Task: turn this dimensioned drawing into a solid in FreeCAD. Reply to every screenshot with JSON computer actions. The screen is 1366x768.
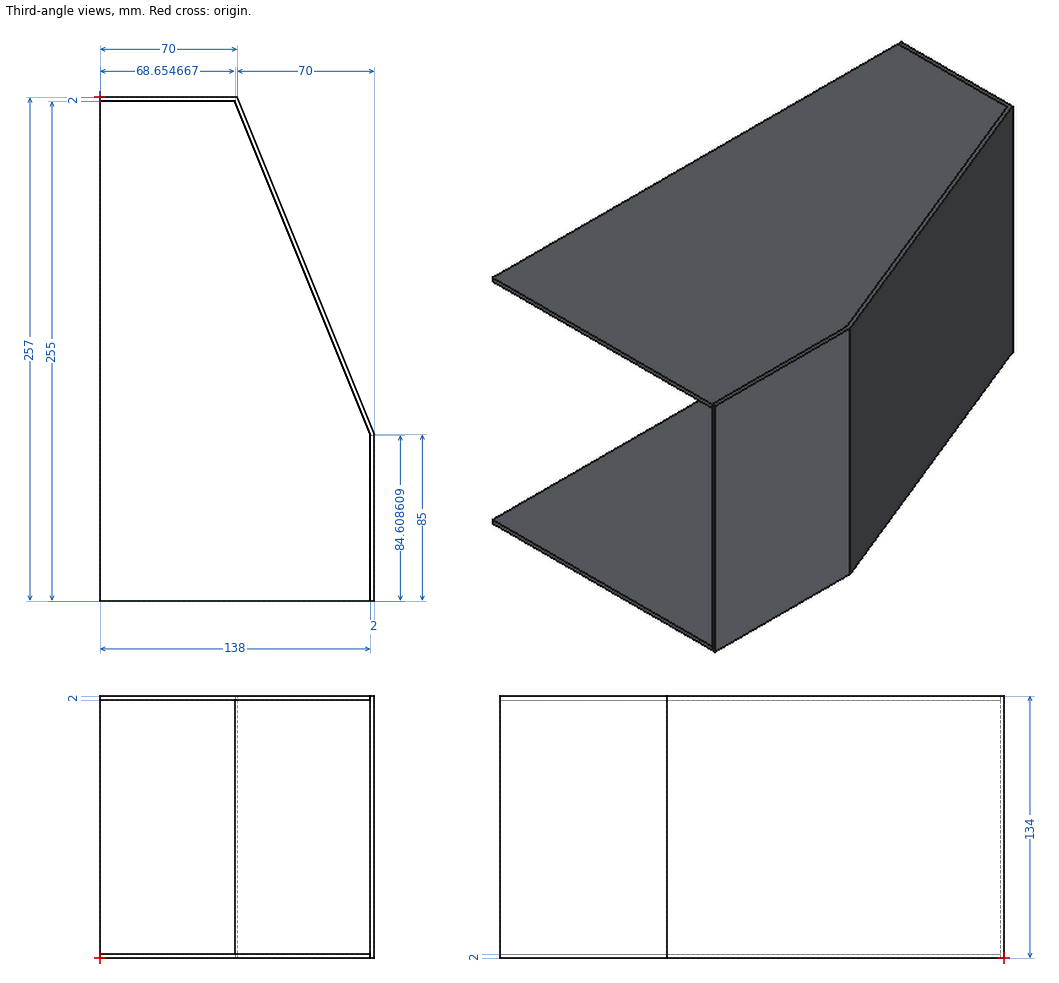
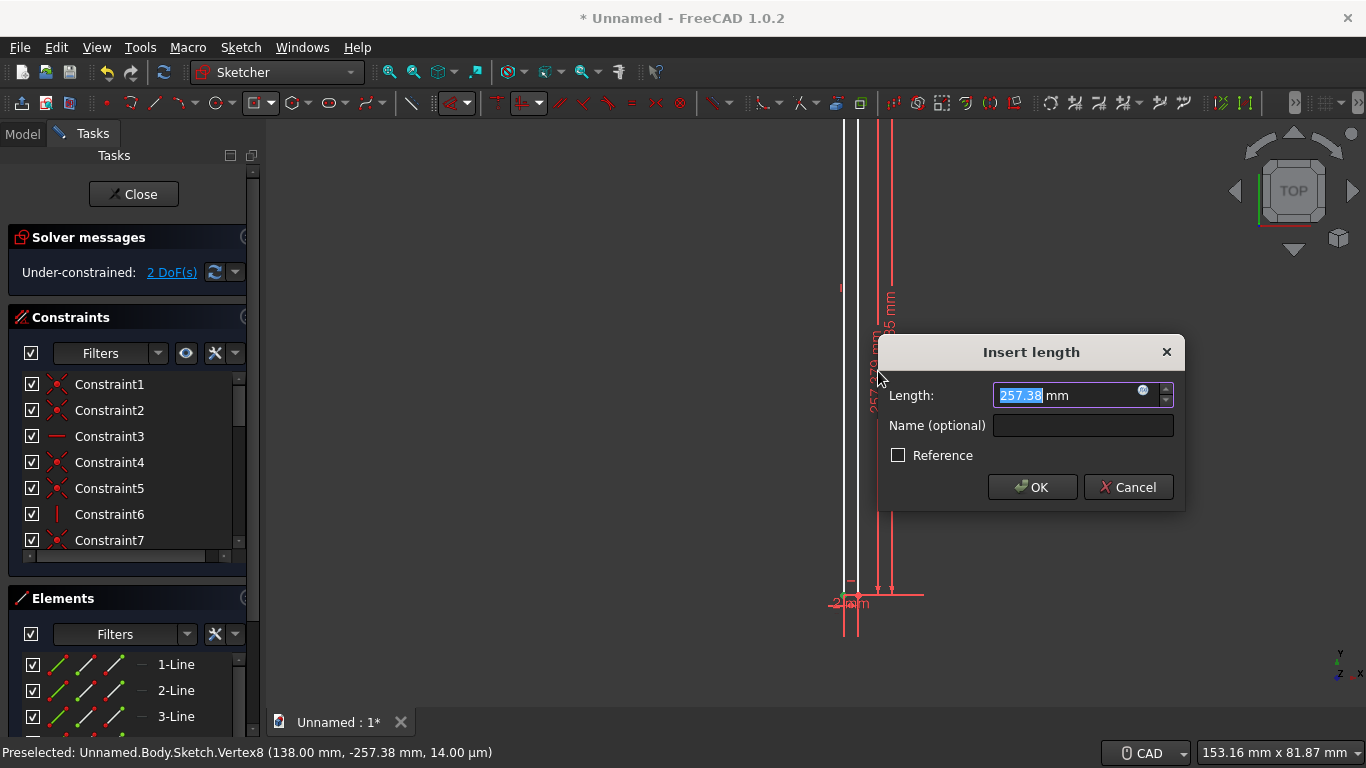
{"action": "type", "text": "257"}
{"action": "key", "text": "Return"}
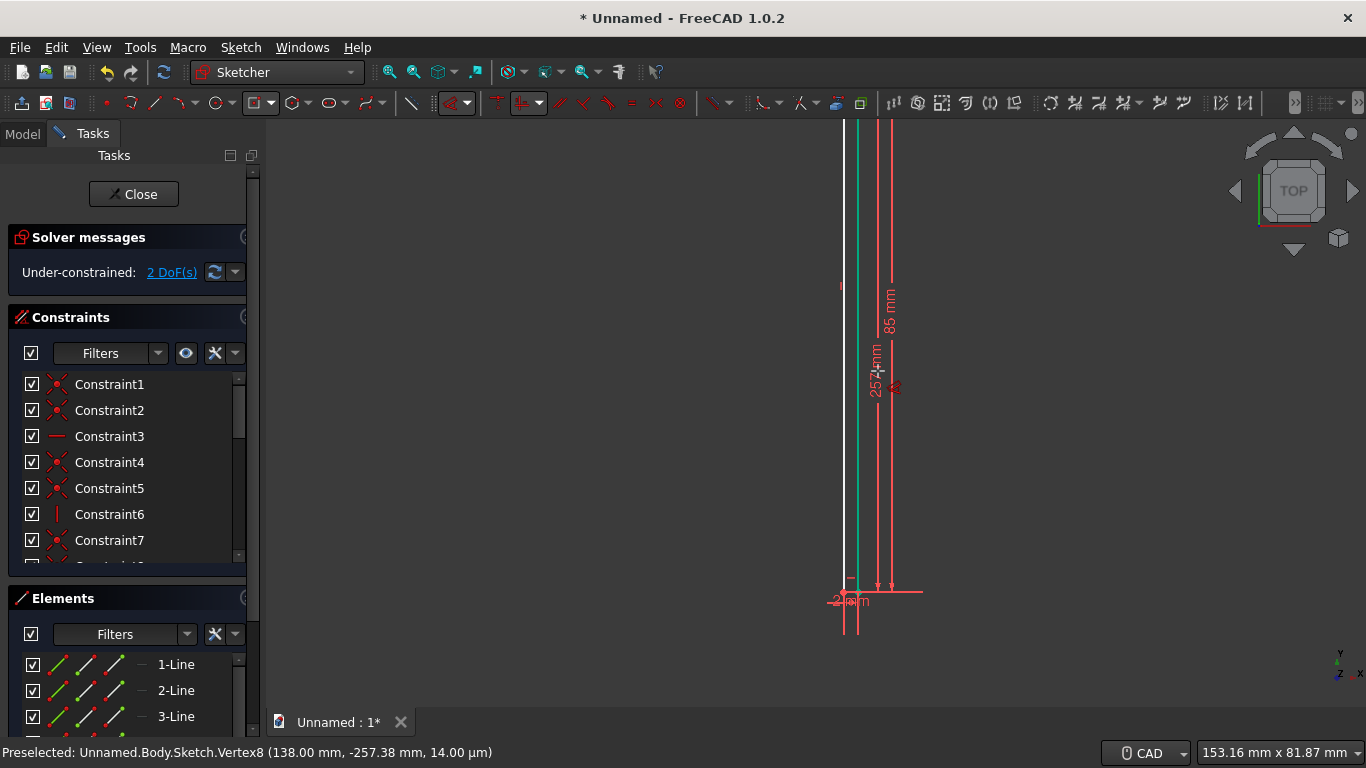
{"action": "scroll", "coordinate": [847, 601], "scroll_direction": "down", "scroll_amount": 8}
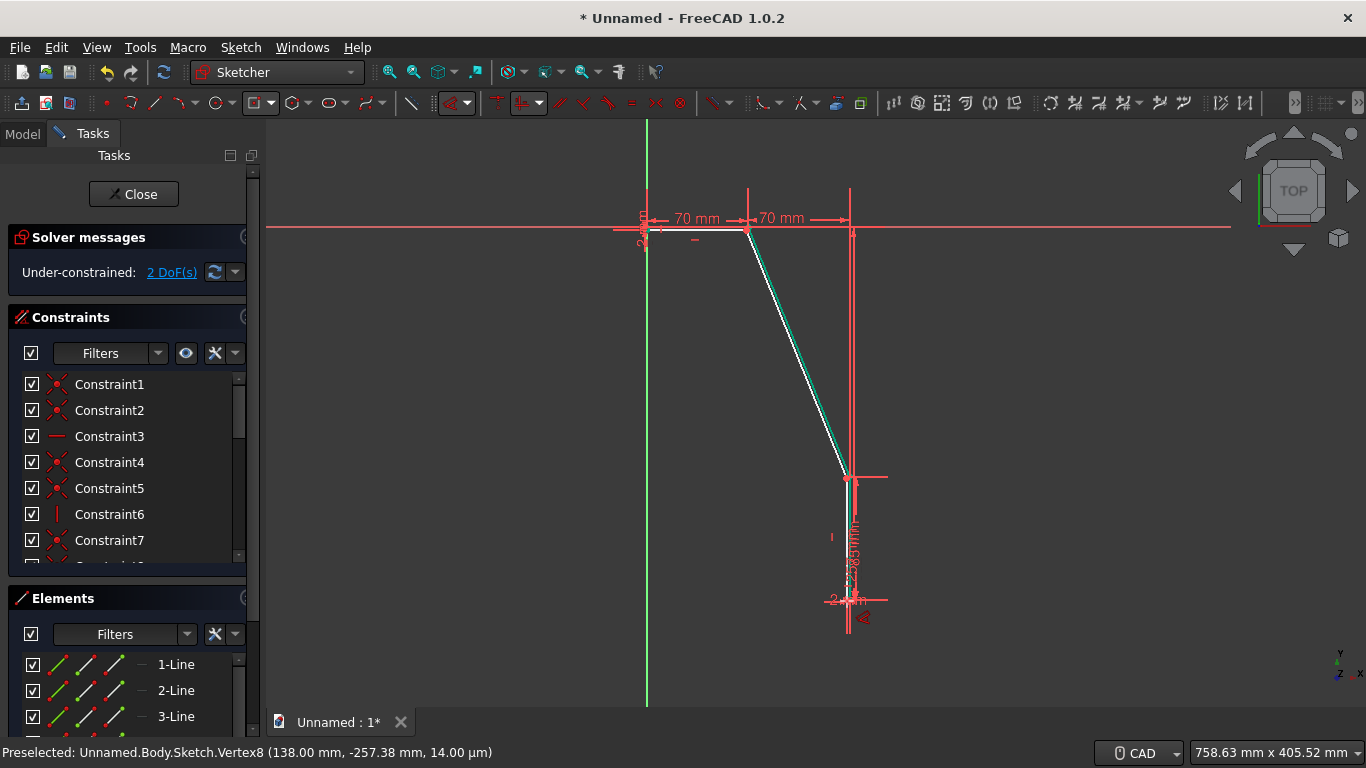
{"action": "scroll", "coordinate": [677, 230], "scroll_direction": "up", "scroll_amount": 8}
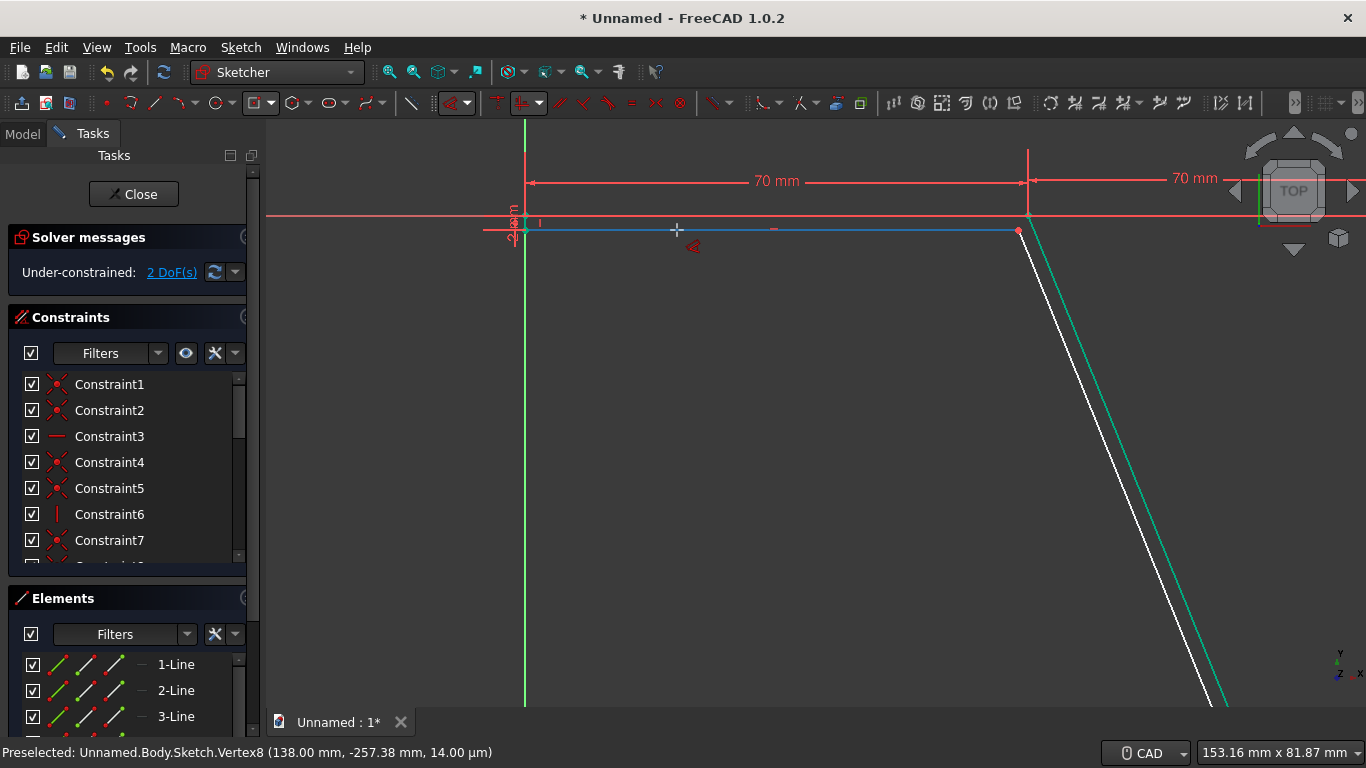
{"action": "left_click", "coordinate": [673, 230]}
{"action": "left_click", "coordinate": [659, 196]}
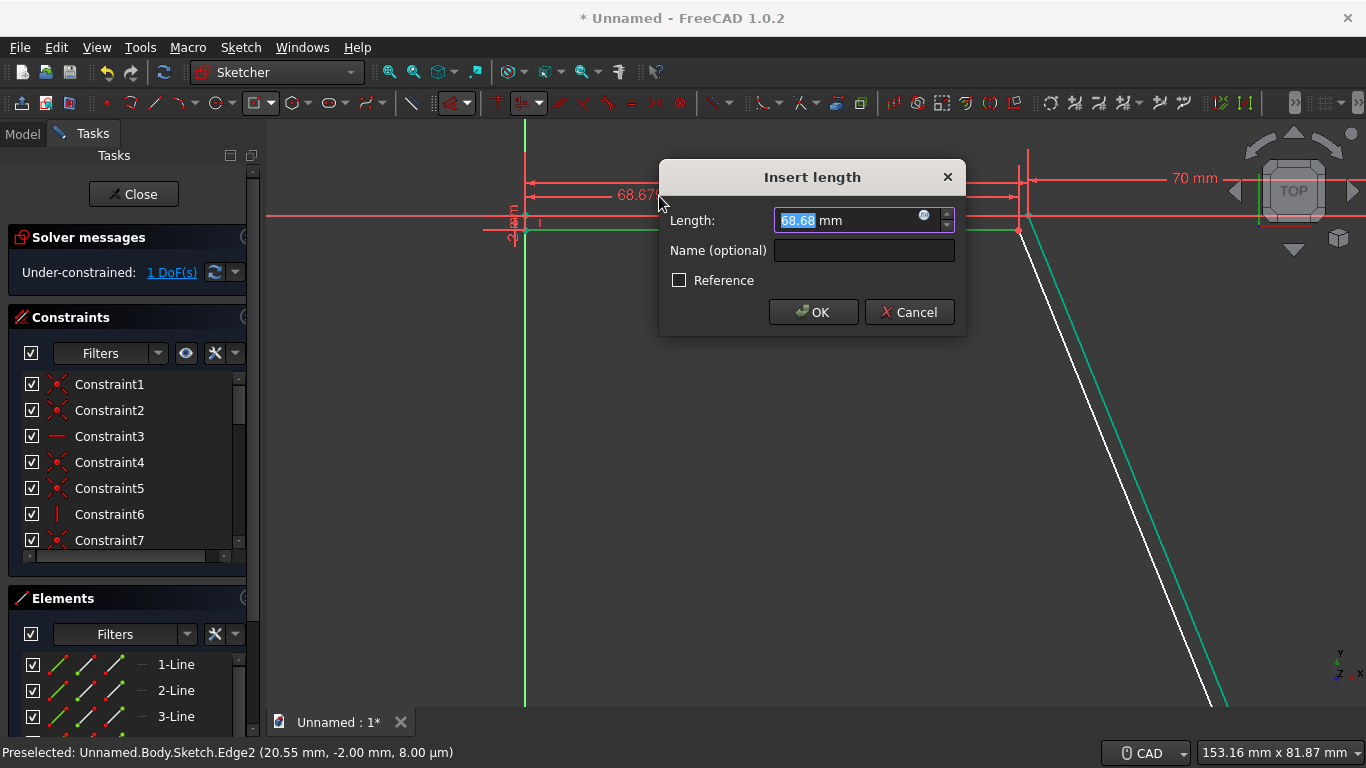
{"action": "type", "text": "68.654667"}
{"action": "key", "text": "Return"}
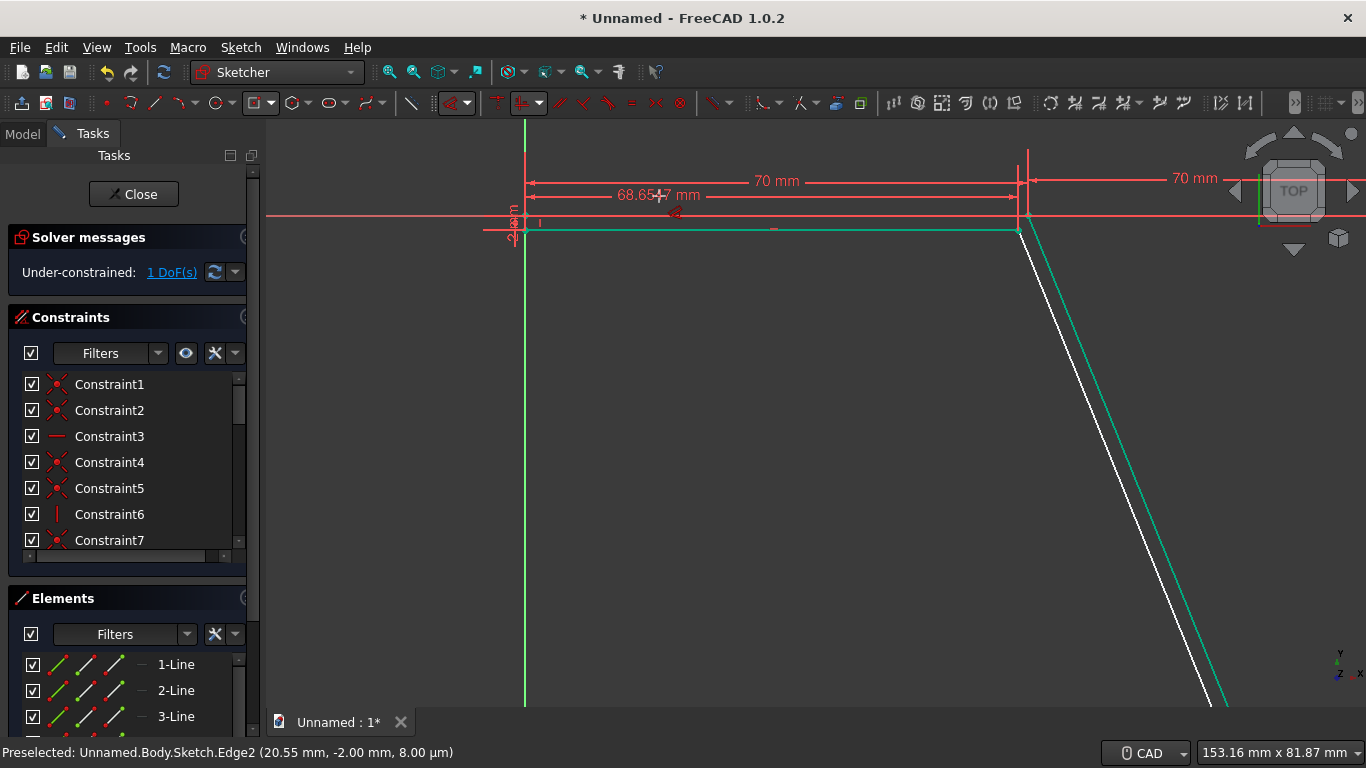
{"action": "scroll", "coordinate": [677, 229], "scroll_direction": "down", "scroll_amount": 8}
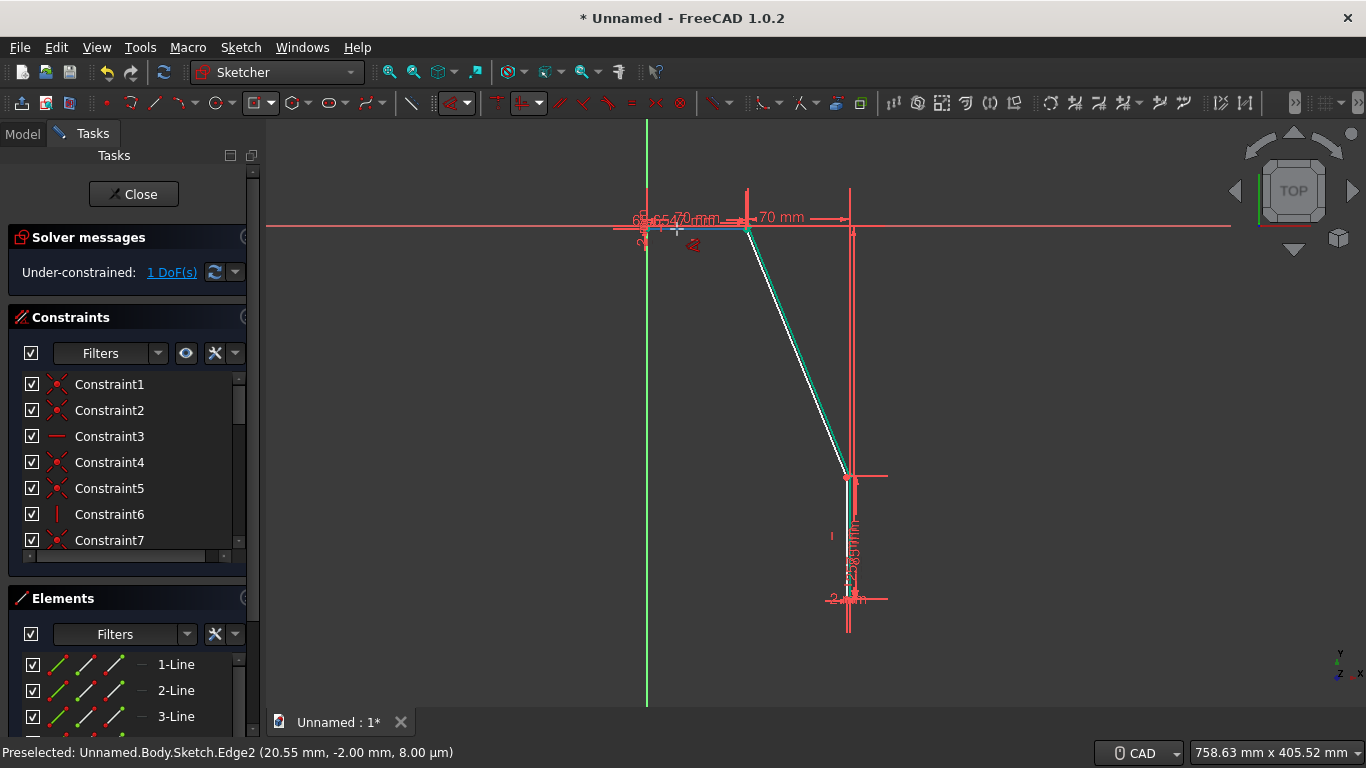
{"action": "scroll", "coordinate": [847, 514], "scroll_direction": "up", "scroll_amount": 8}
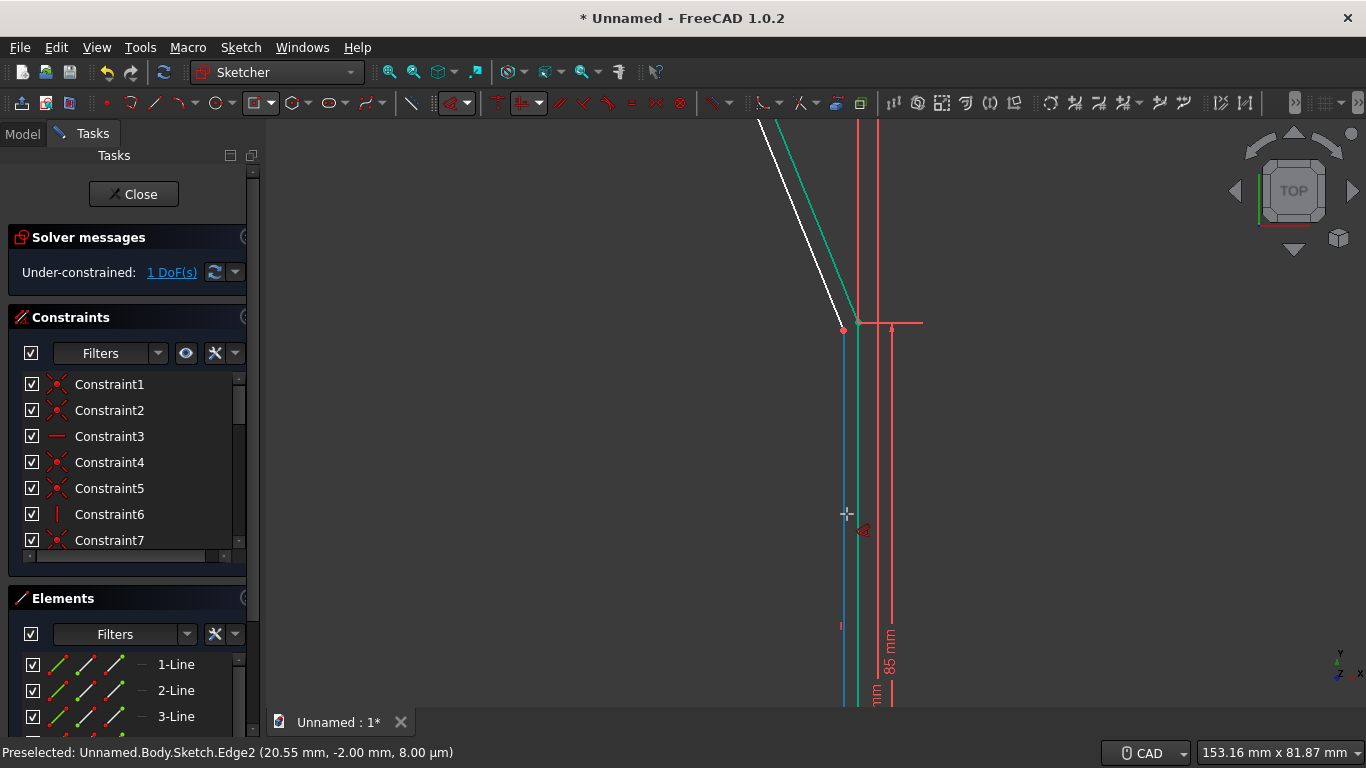
{"action": "left_click", "coordinate": [844, 511]}
{"action": "left_click", "coordinate": [878, 505]}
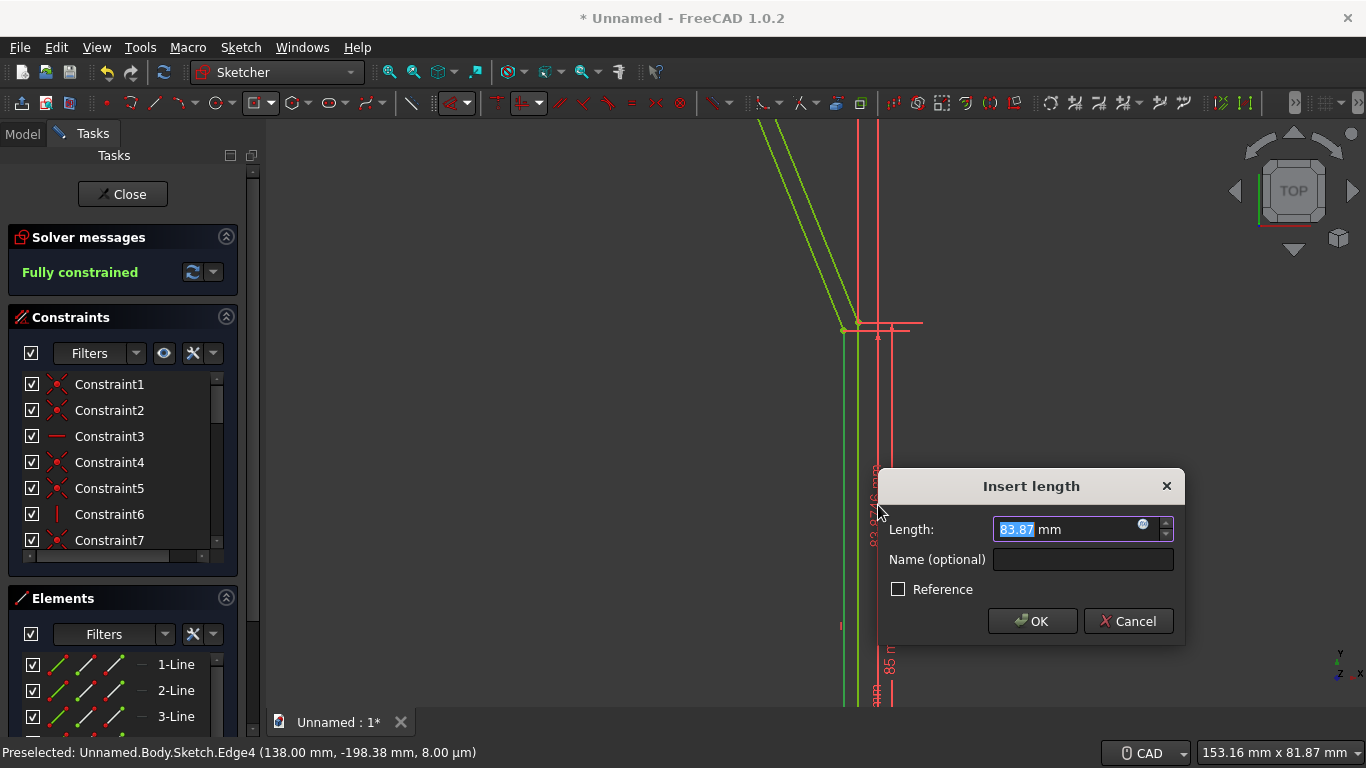
{"action": "type", "text": "84.608609"}
{"action": "key", "text": "Return"}
{"action": "key", "text": "Escape"}